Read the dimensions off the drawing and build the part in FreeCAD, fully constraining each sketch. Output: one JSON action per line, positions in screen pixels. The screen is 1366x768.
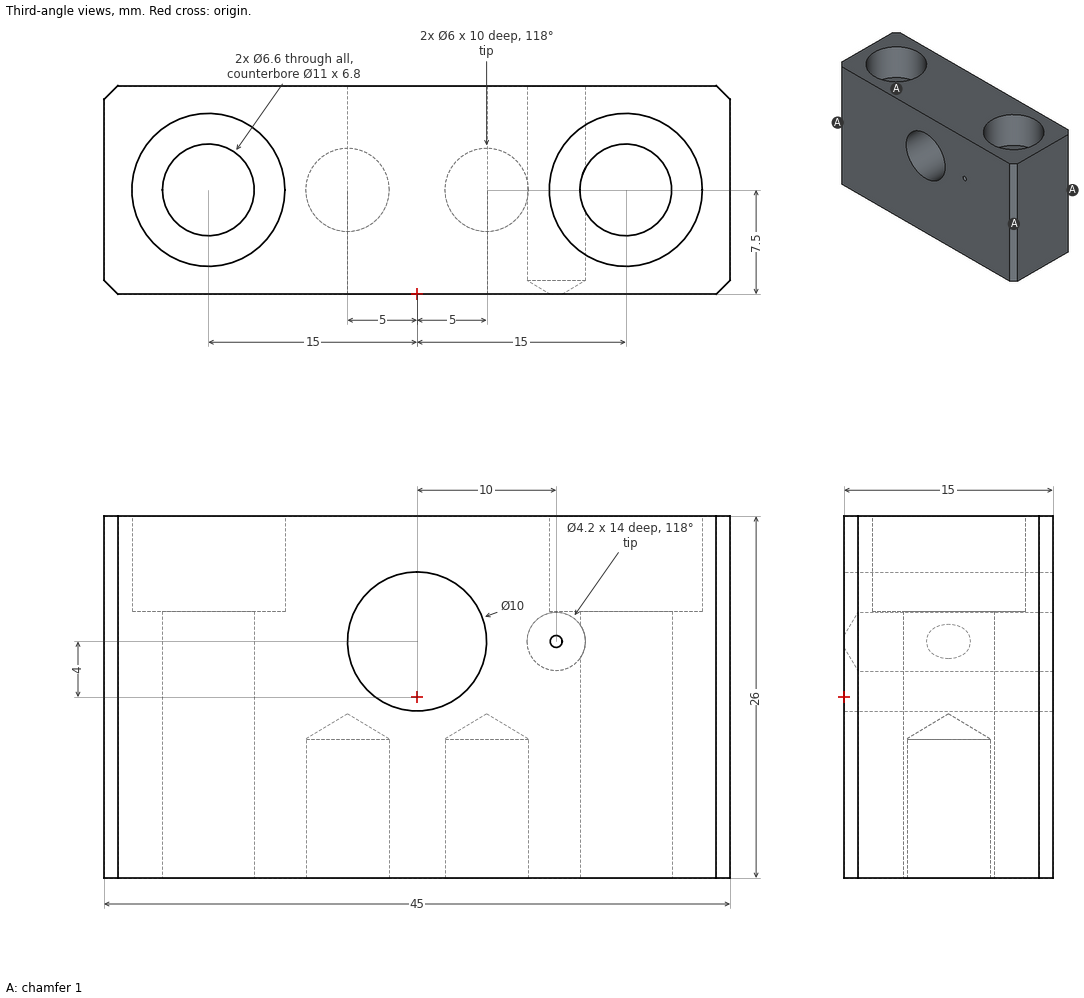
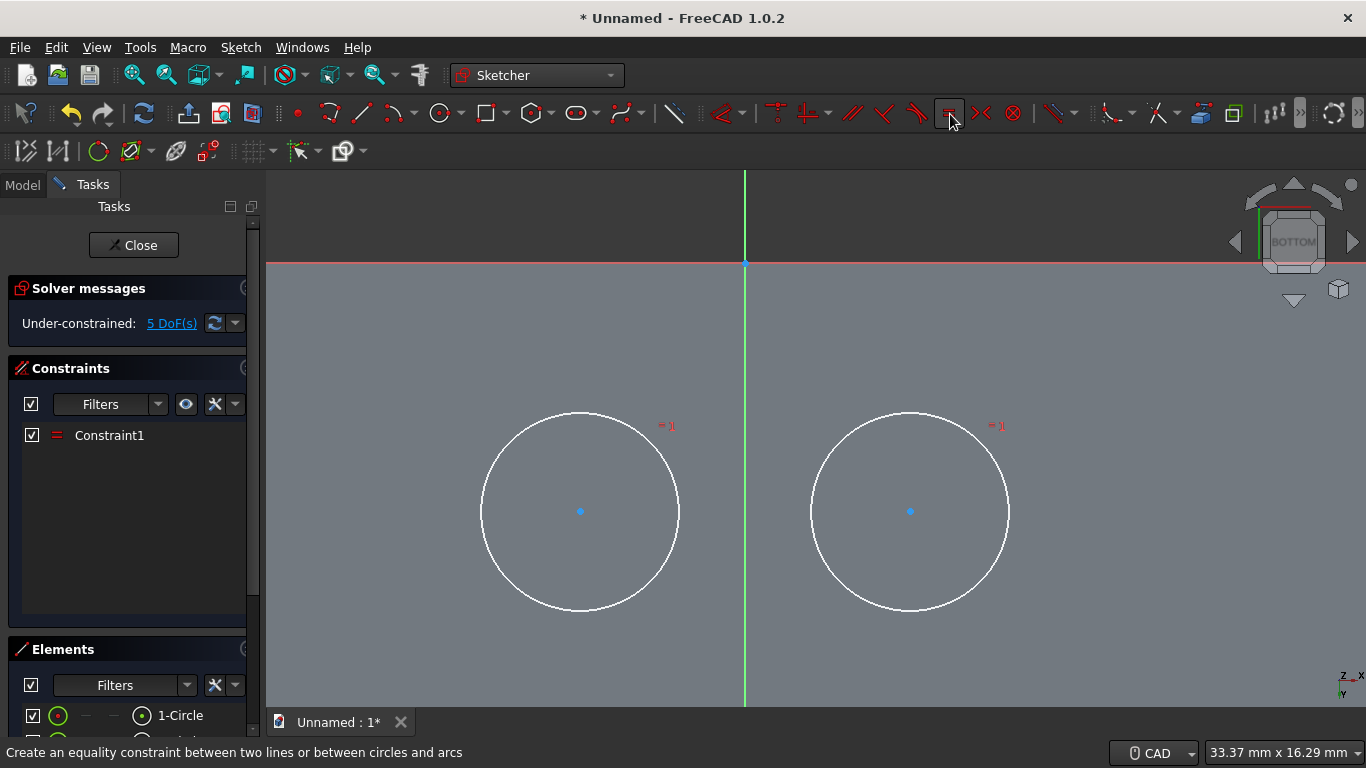
{"action": "left_click", "coordinate": [910, 512]}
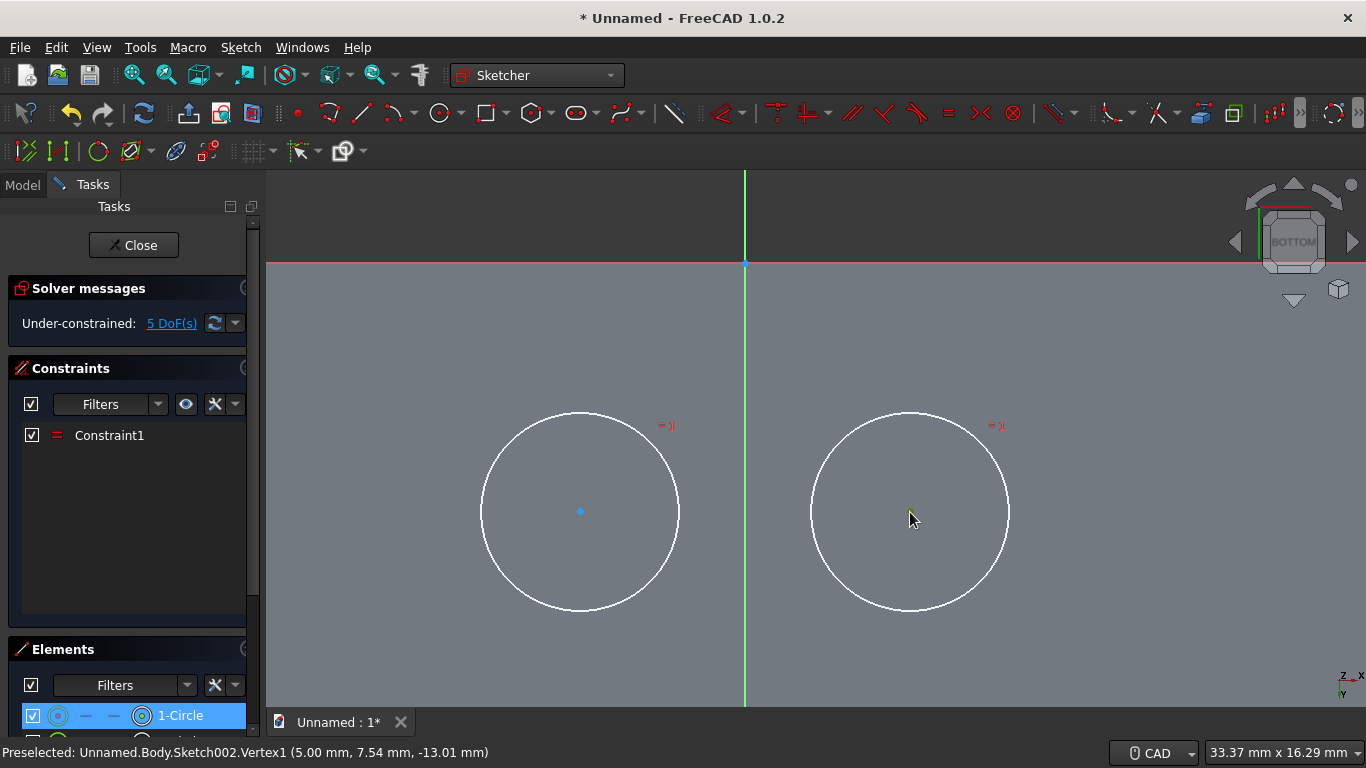
{"action": "left_click", "coordinate": [580, 512]}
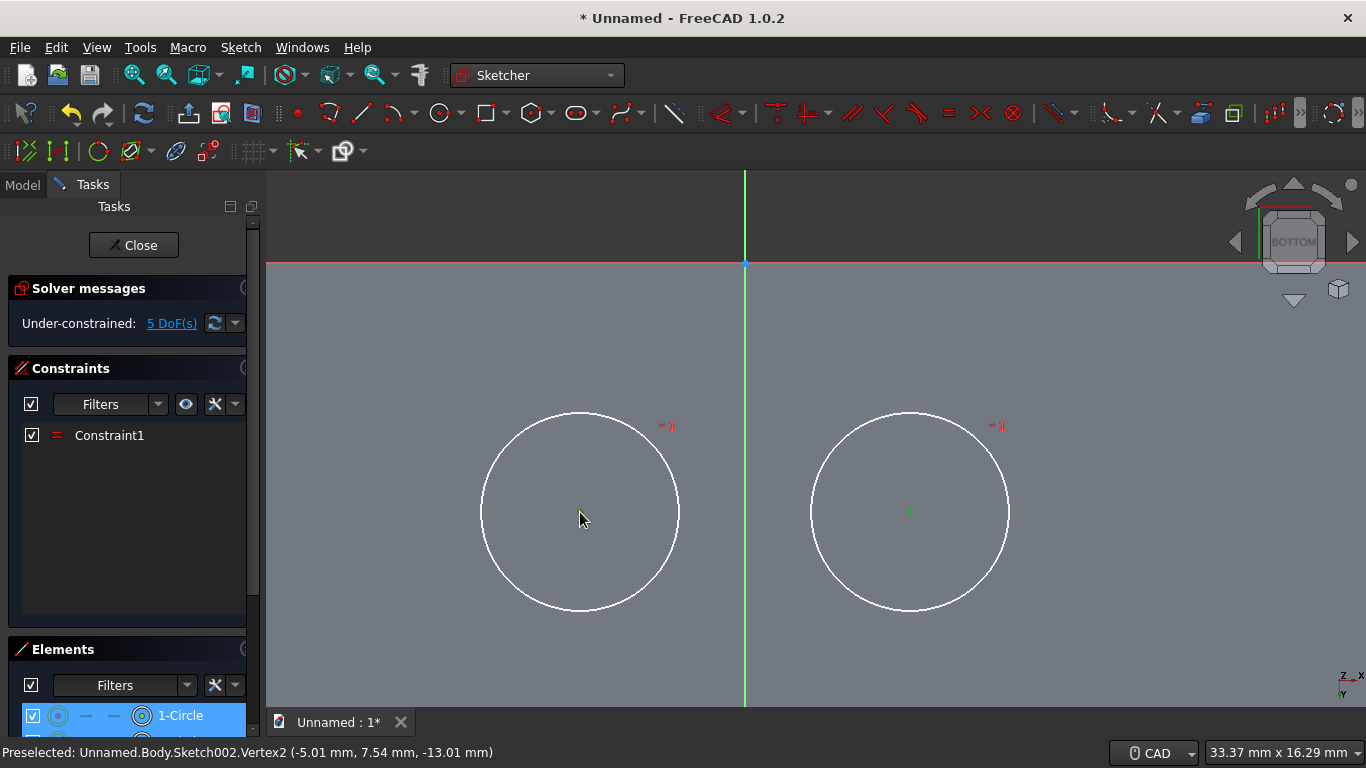
{"action": "key", "text": "h"}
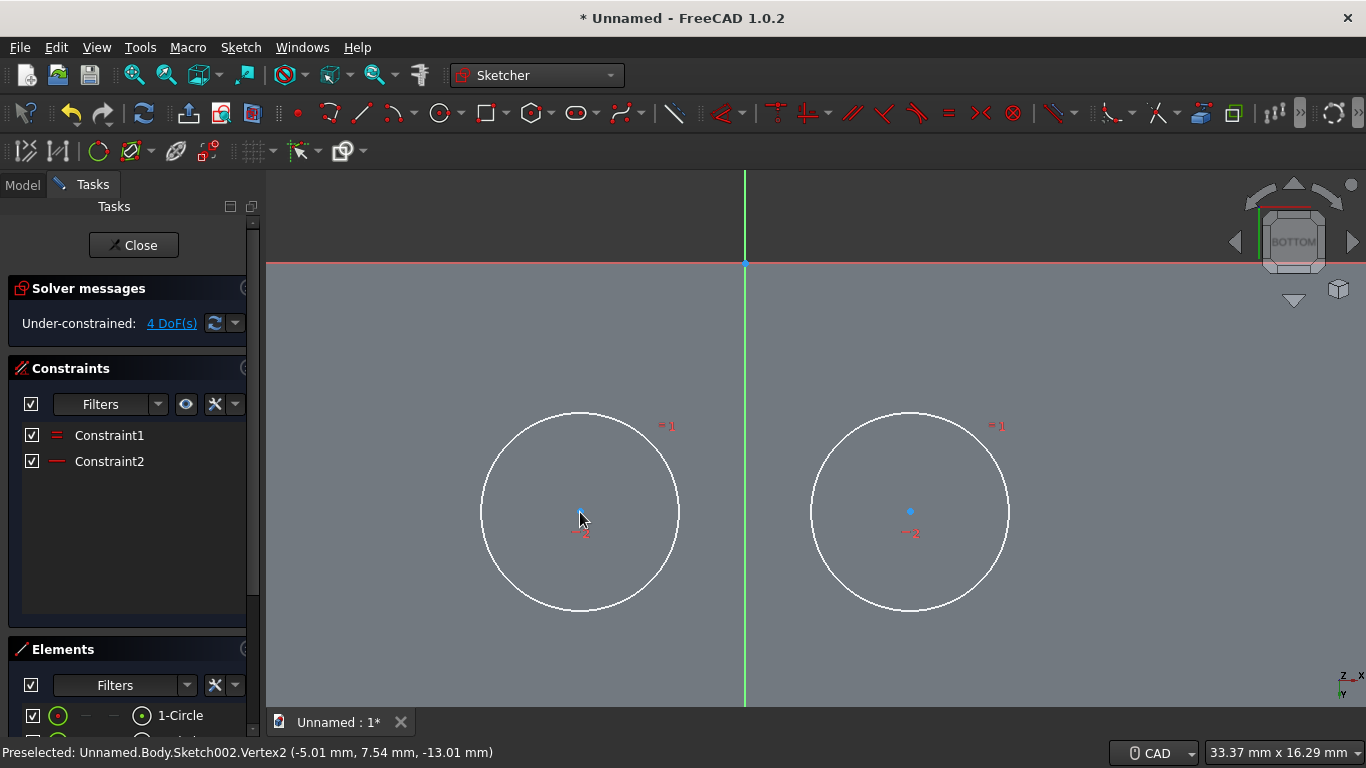
{"action": "left_click", "coordinate": [722, 114]}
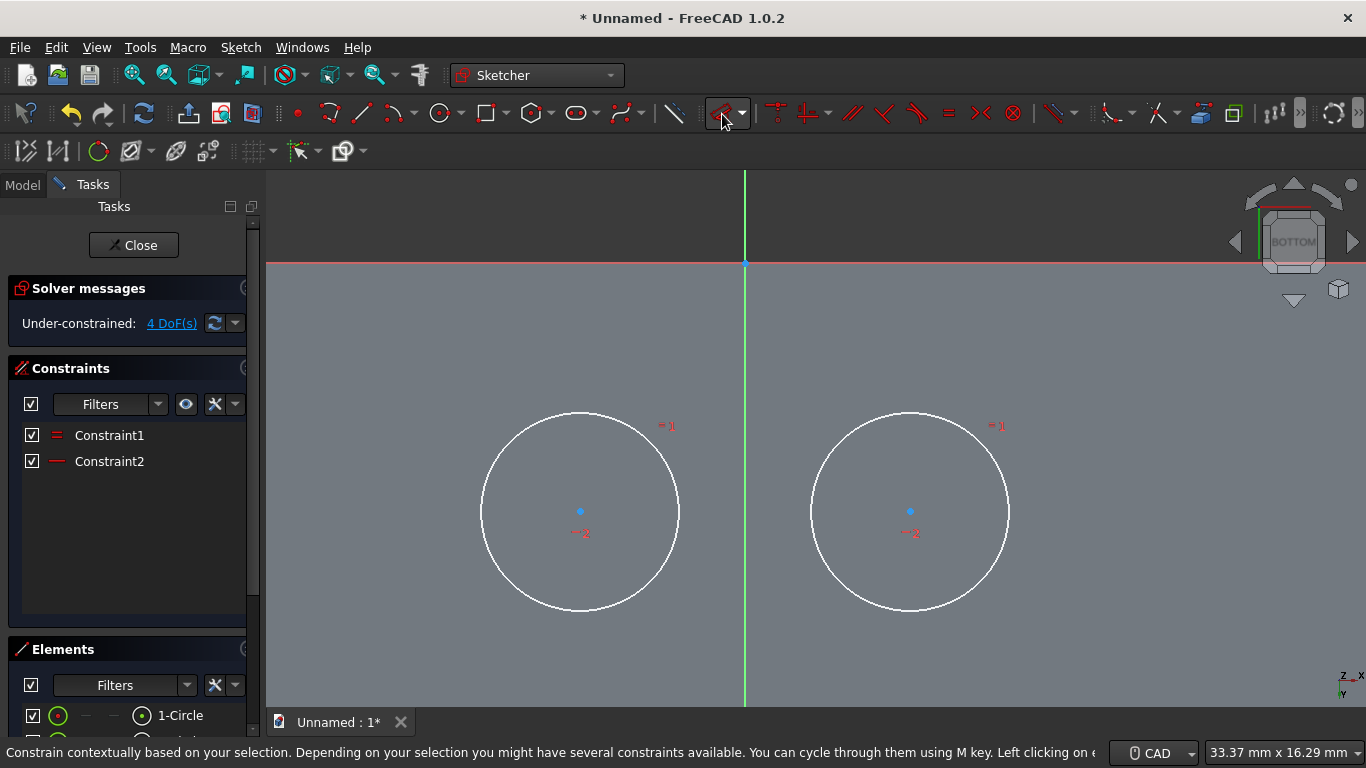
{"action": "left_click", "coordinate": [980, 442]}
{"action": "left_click", "coordinate": [1003, 419]}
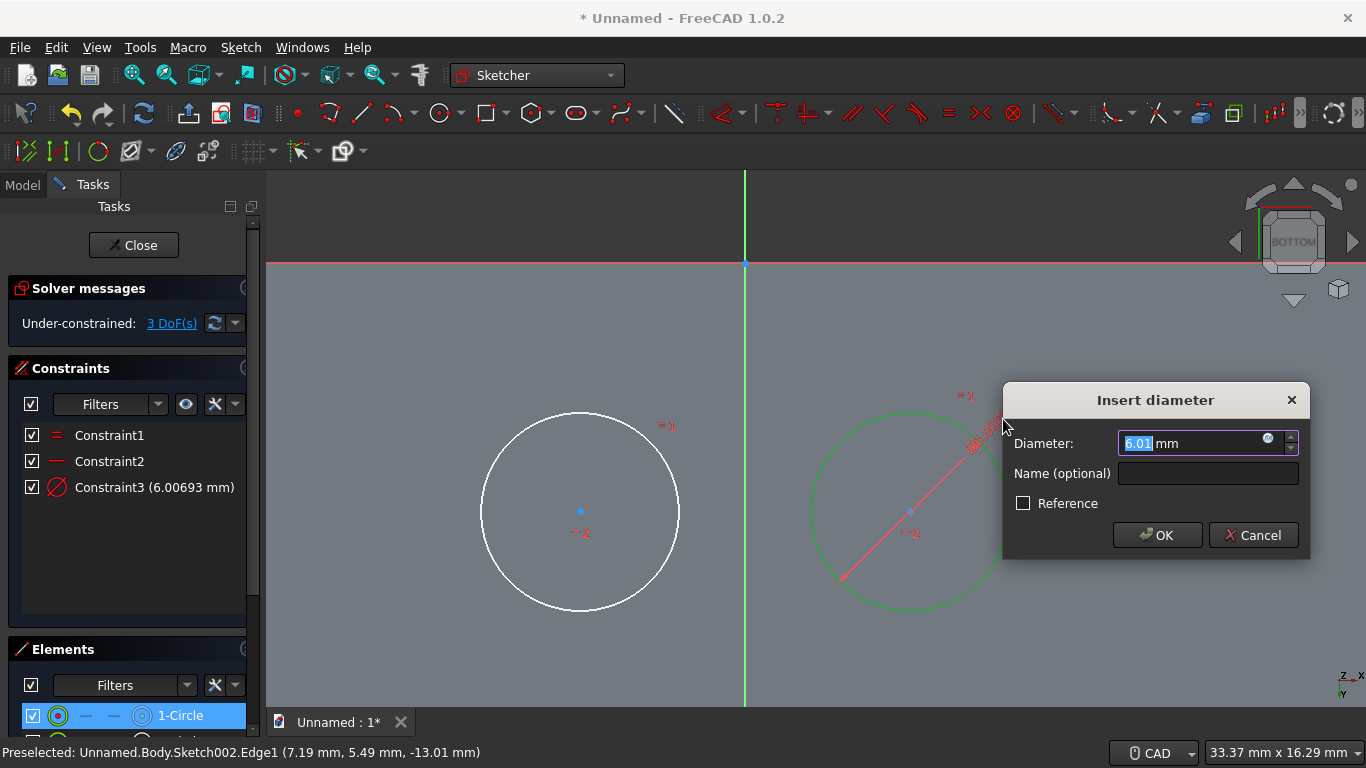
{"action": "type", "text": "6"}
{"action": "key", "text": "Return"}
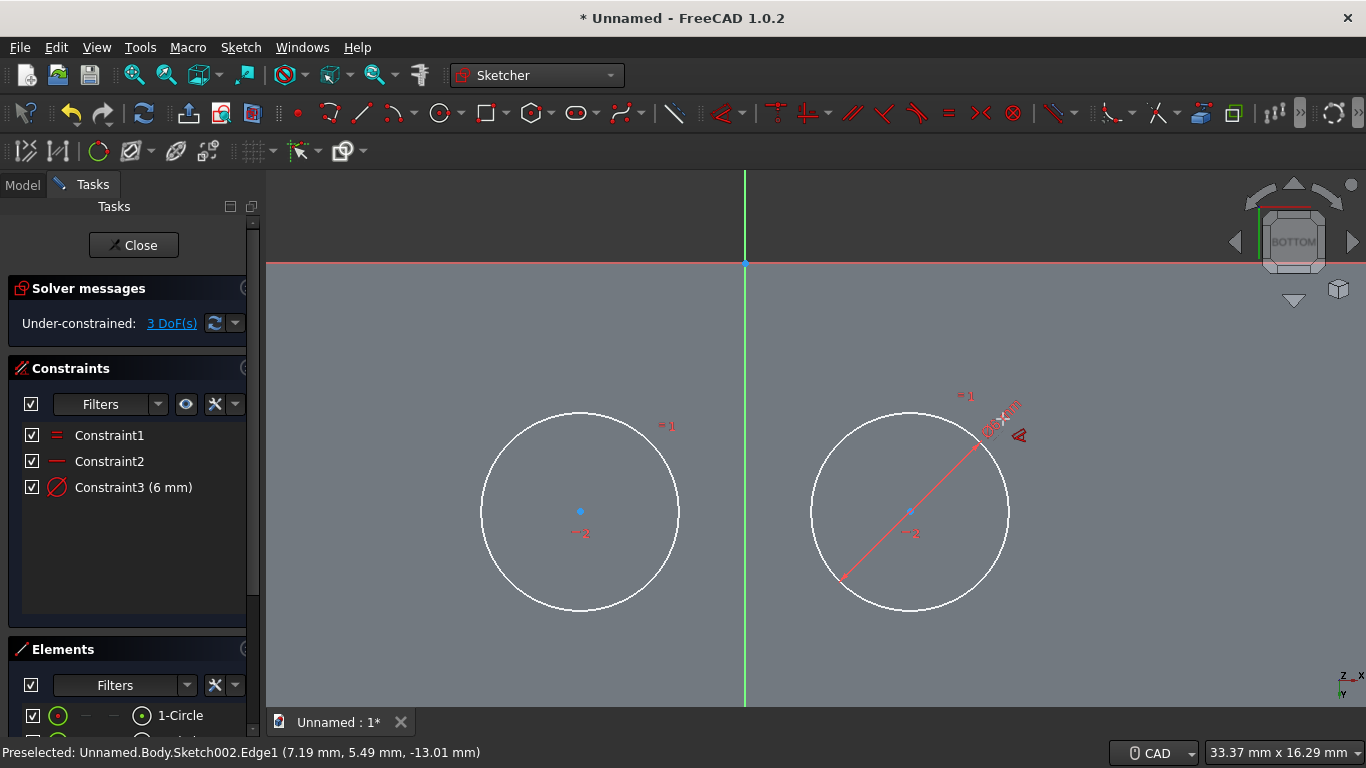
{"action": "left_click", "coordinate": [910, 512]}
{"action": "left_click", "coordinate": [828, 229]}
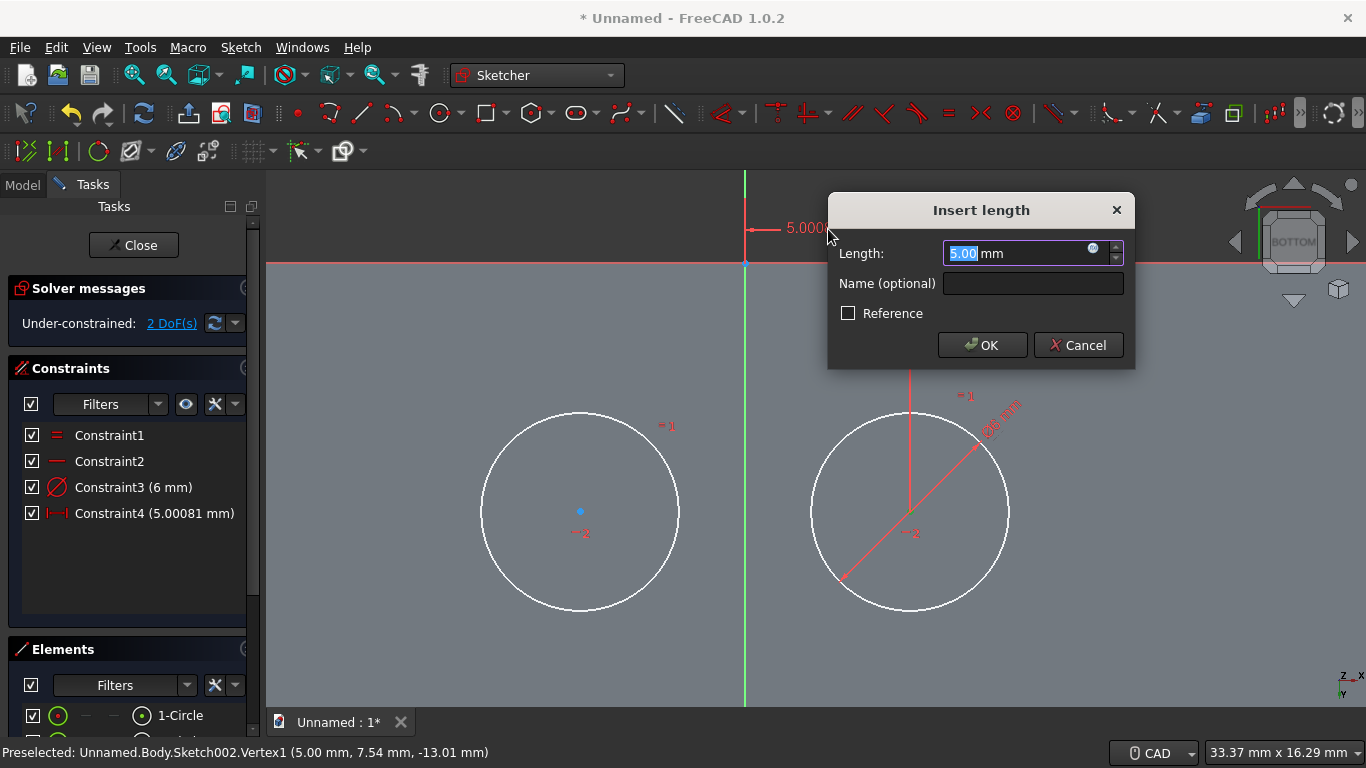
{"action": "type", "text": "5"}
{"action": "key", "text": "Return"}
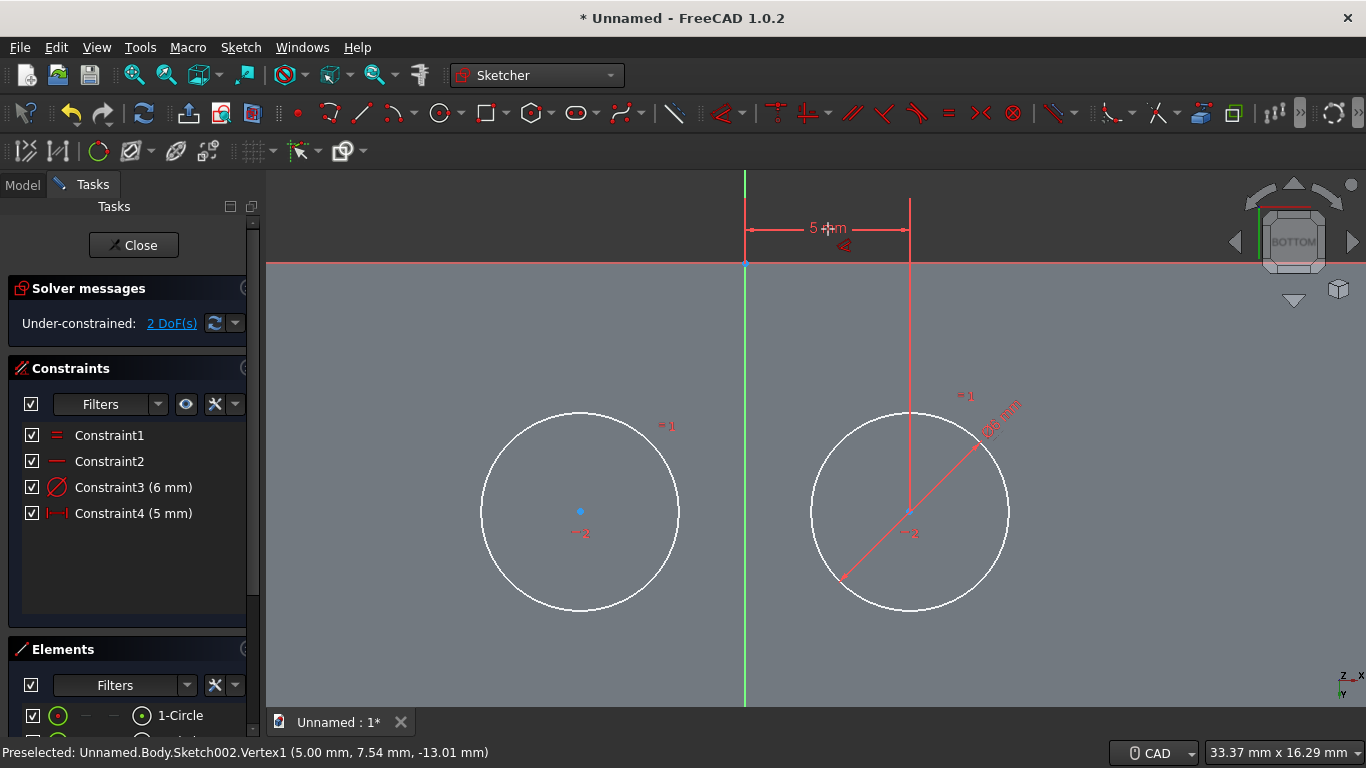
{"action": "left_click", "coordinate": [580, 512]}
{"action": "left_click", "coordinate": [663, 229]}